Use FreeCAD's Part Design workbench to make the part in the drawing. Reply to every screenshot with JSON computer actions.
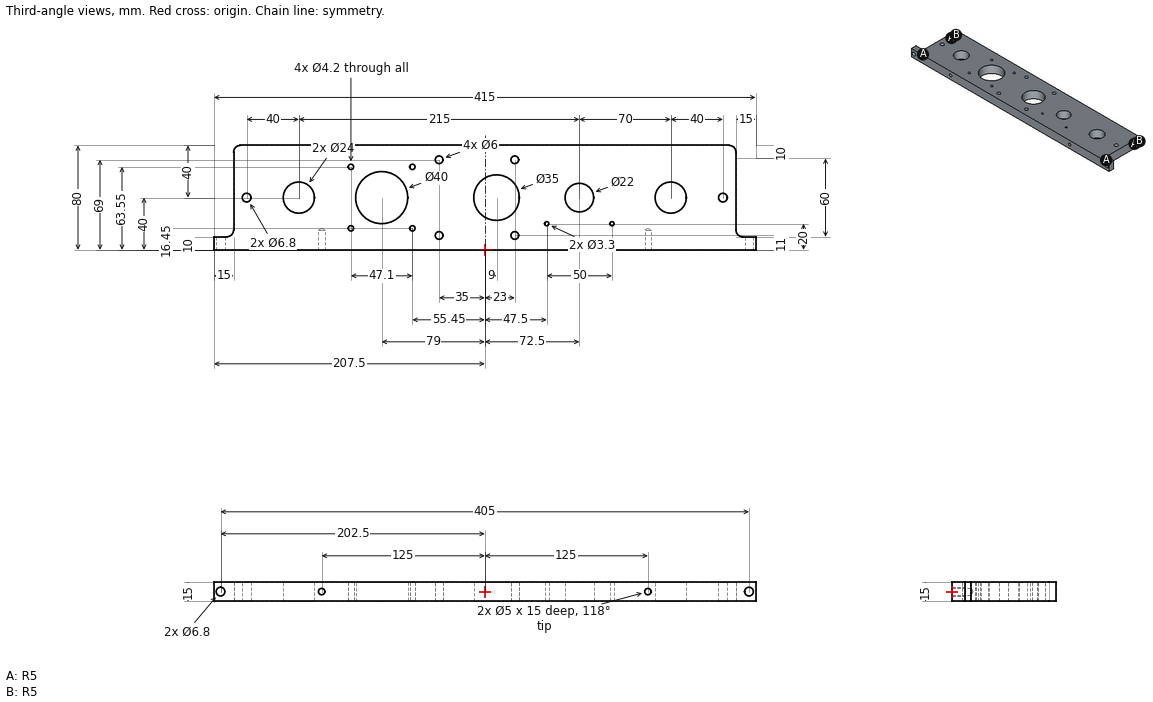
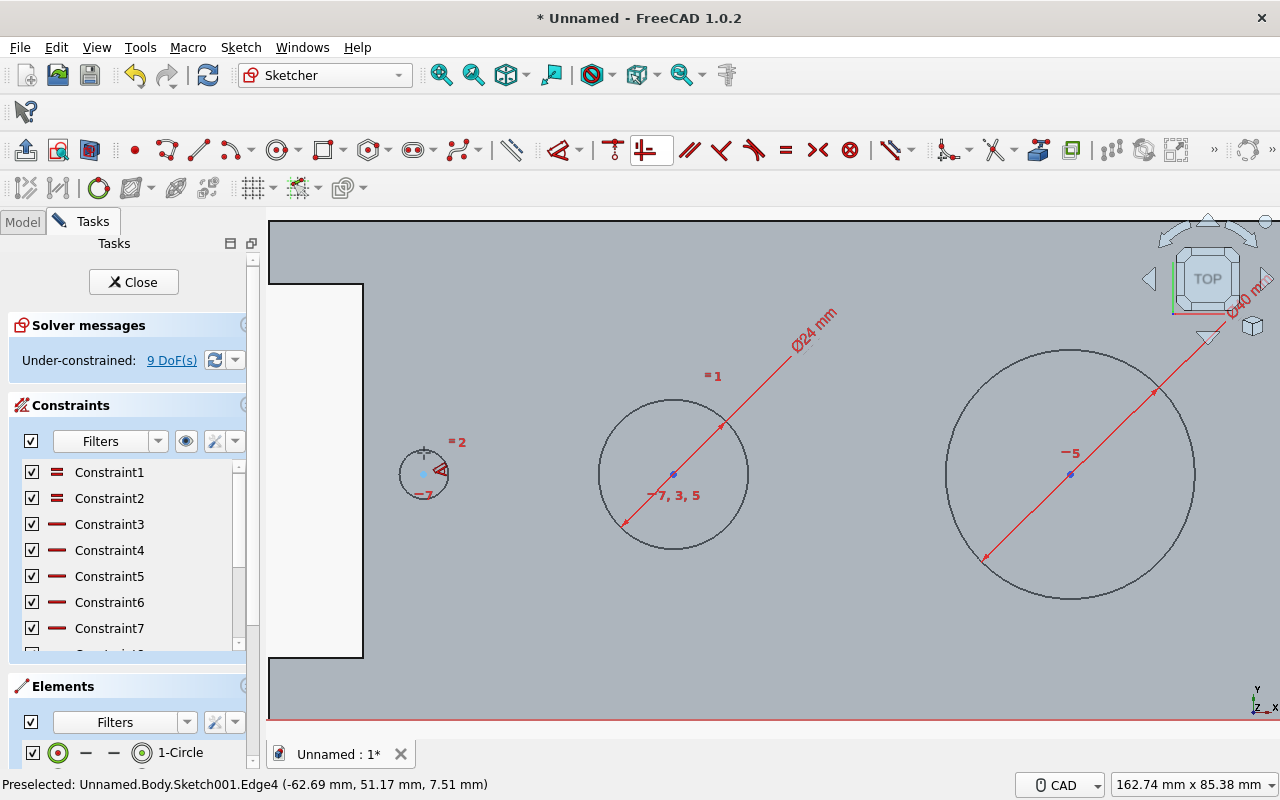
{"action": "left_click", "coordinate": [425, 450]}
{"action": "left_click", "coordinate": [426, 418]}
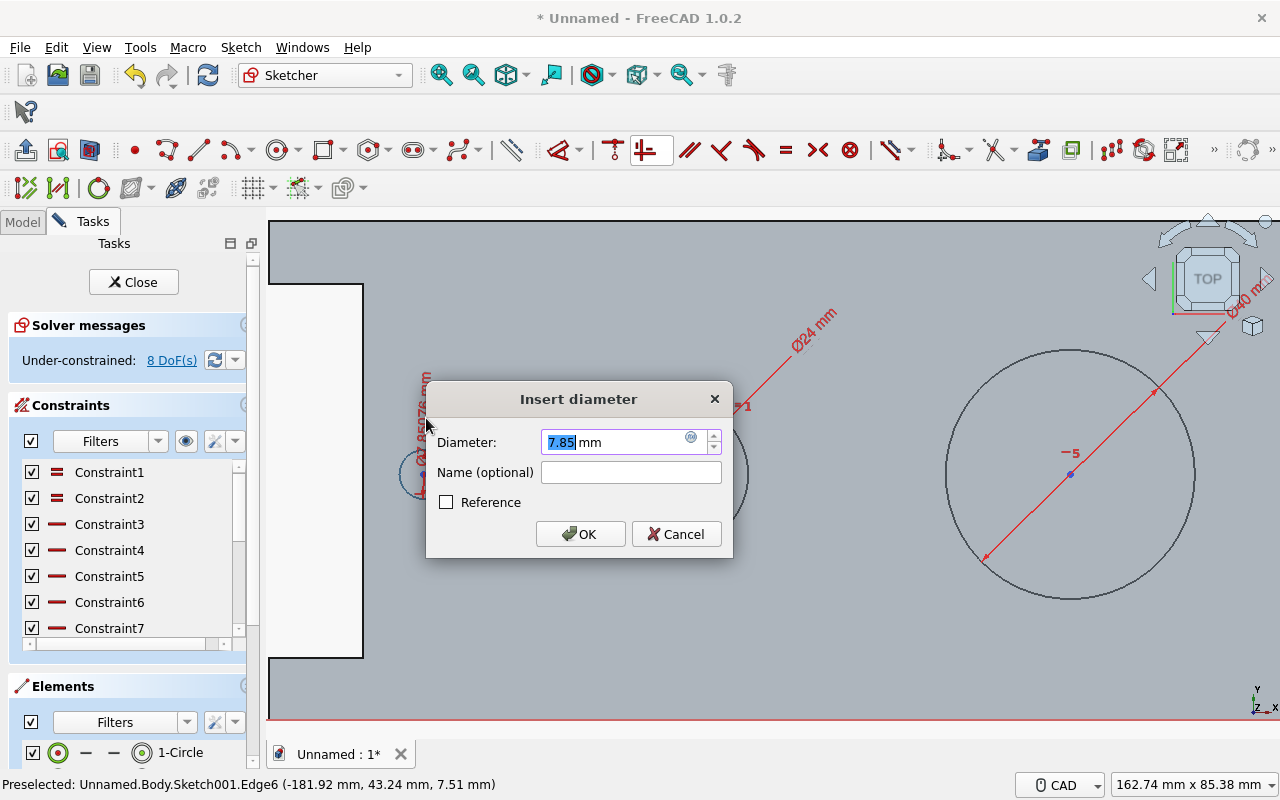
{"action": "type", "text": "6.8"}
{"action": "key", "text": "Return"}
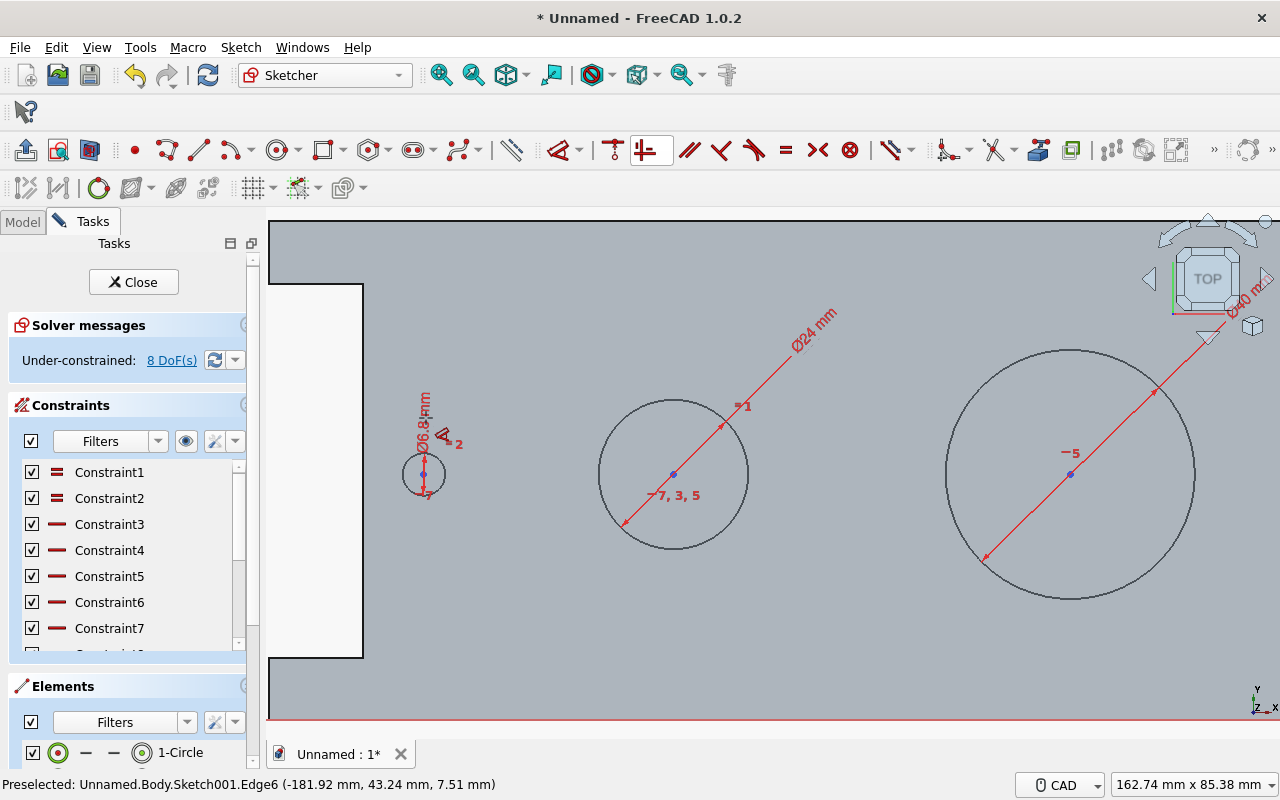
{"action": "scroll", "coordinate": [424, 453], "scroll_direction": "down", "scroll_amount": 7}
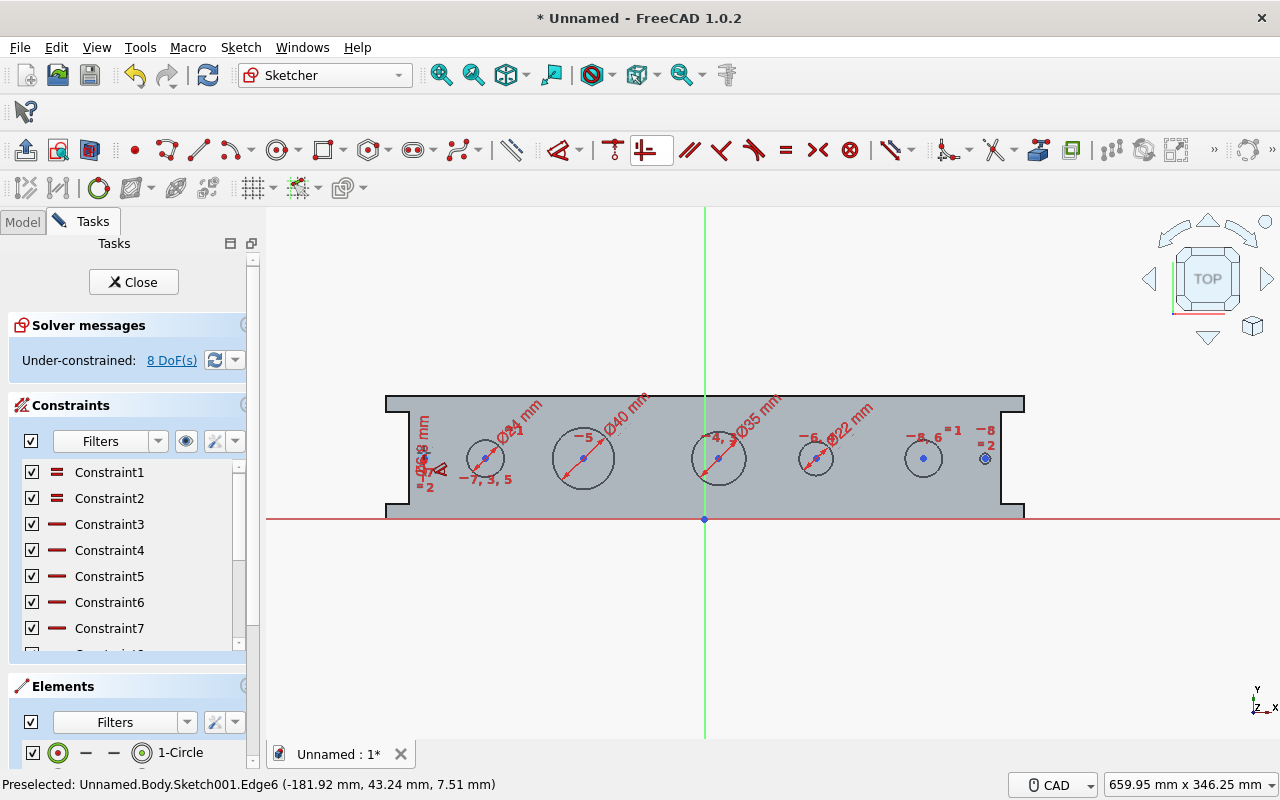
{"action": "scroll", "coordinate": [719, 459], "scroll_direction": "up", "scroll_amount": 6}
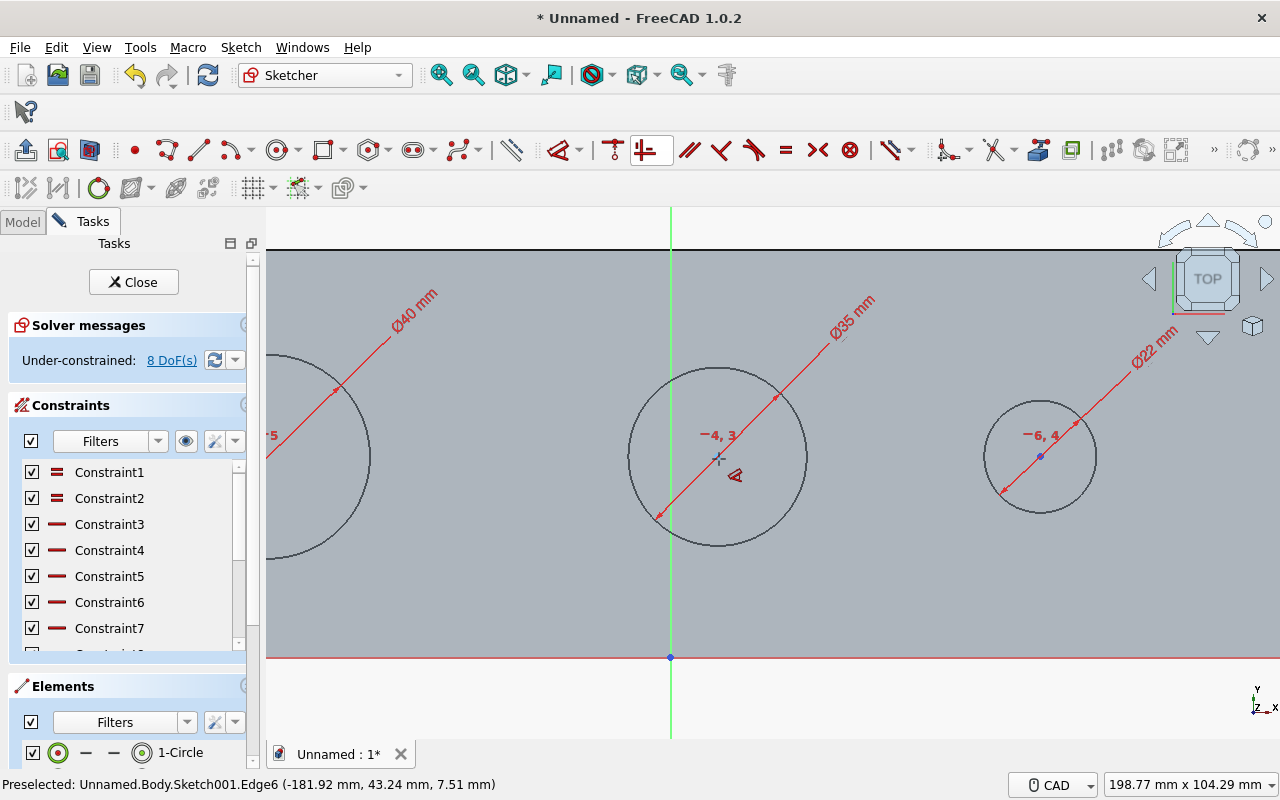
{"action": "left_click", "coordinate": [718, 457]}
{"action": "left_click", "coordinate": [694, 692]}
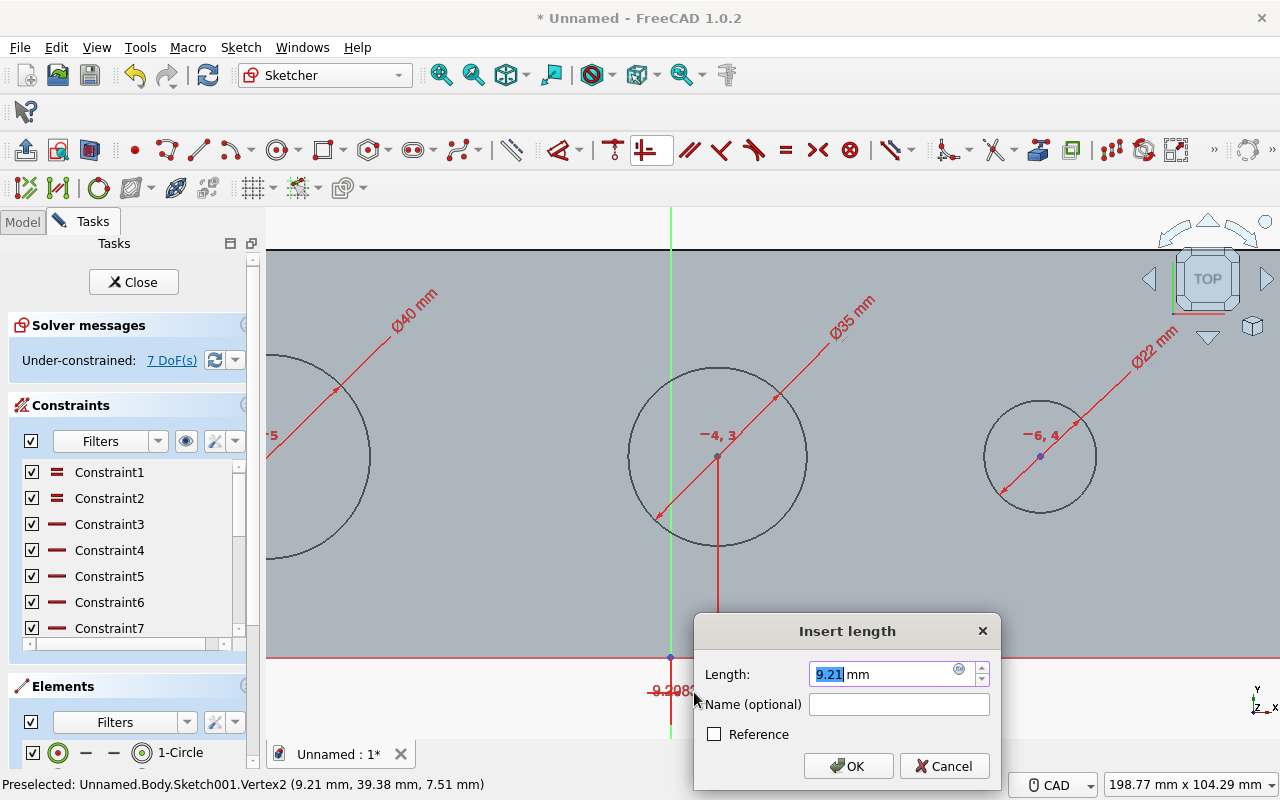
{"action": "type", "text": "9"}
{"action": "key", "text": "Return"}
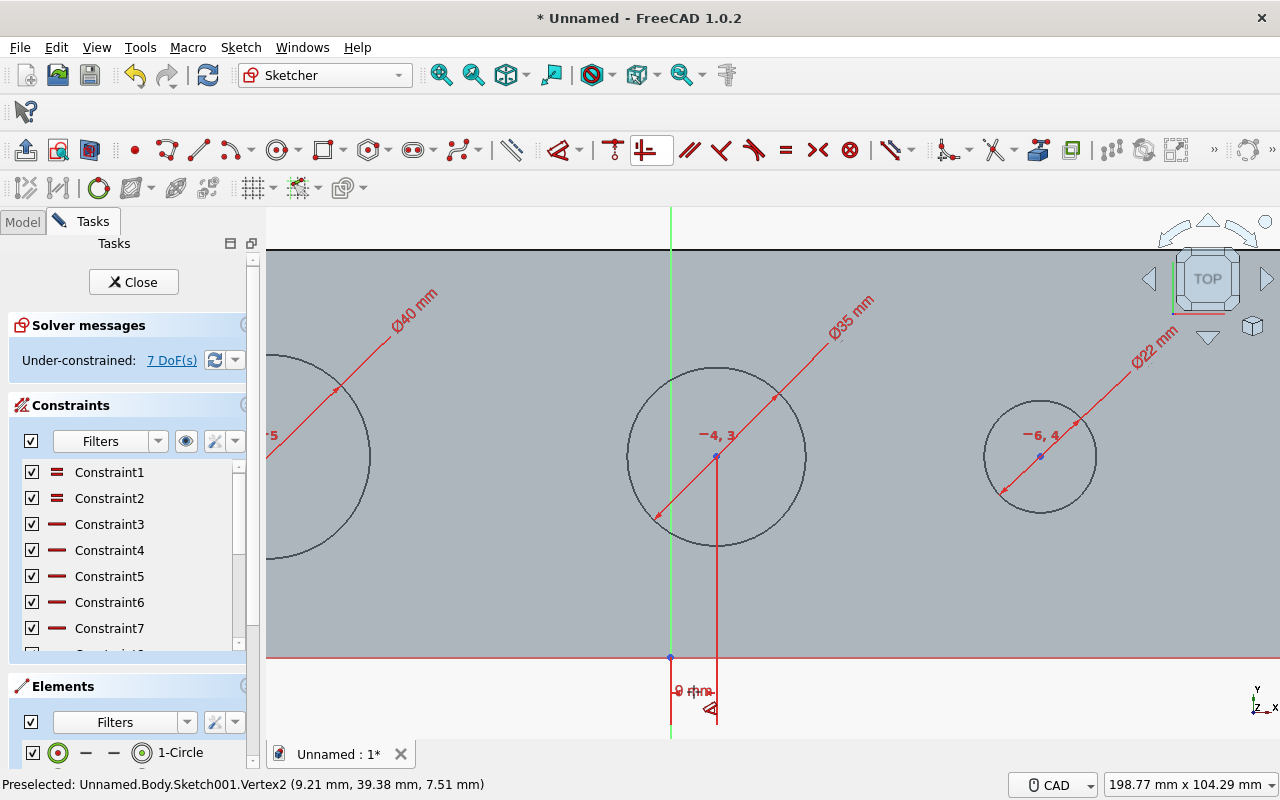
{"action": "scroll", "coordinate": [719, 459], "scroll_direction": "down", "scroll_amount": 6}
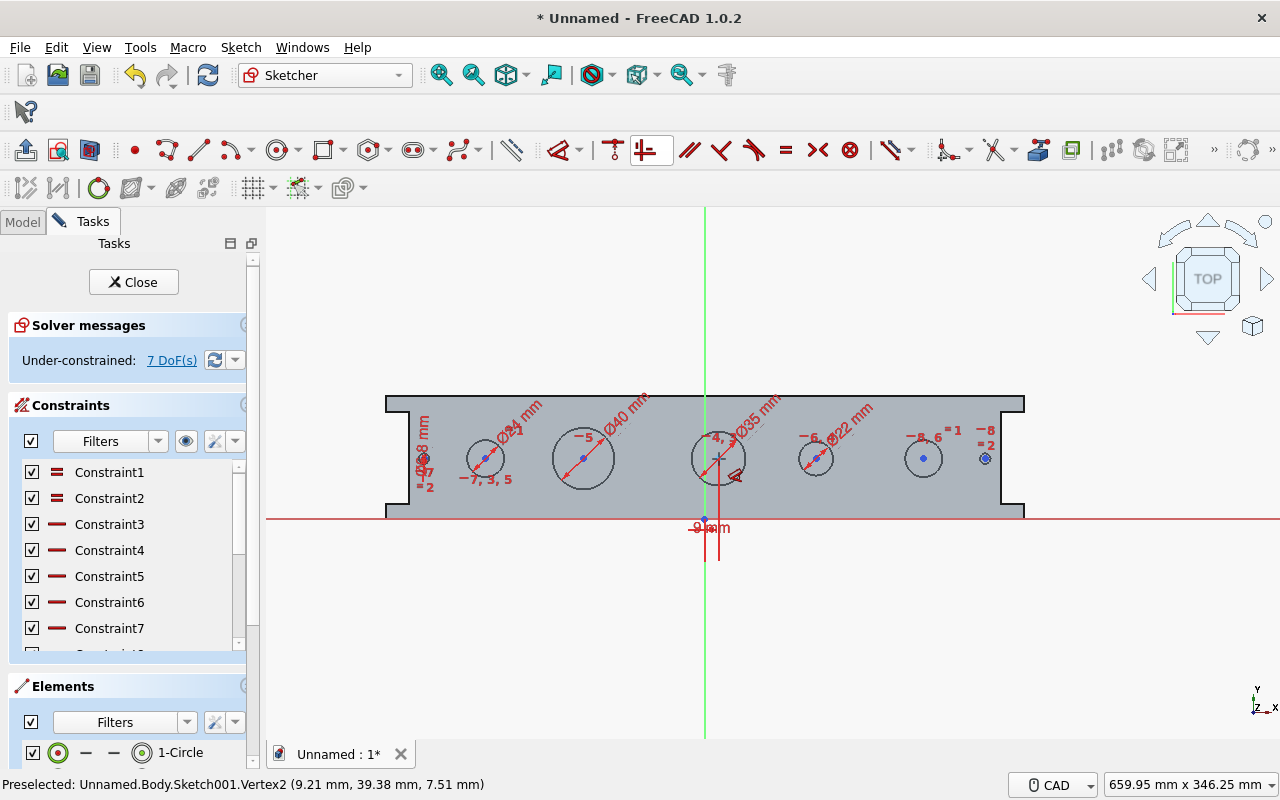
{"action": "left_click", "coordinate": [486, 459]}
{"action": "left_click", "coordinate": [452, 489]}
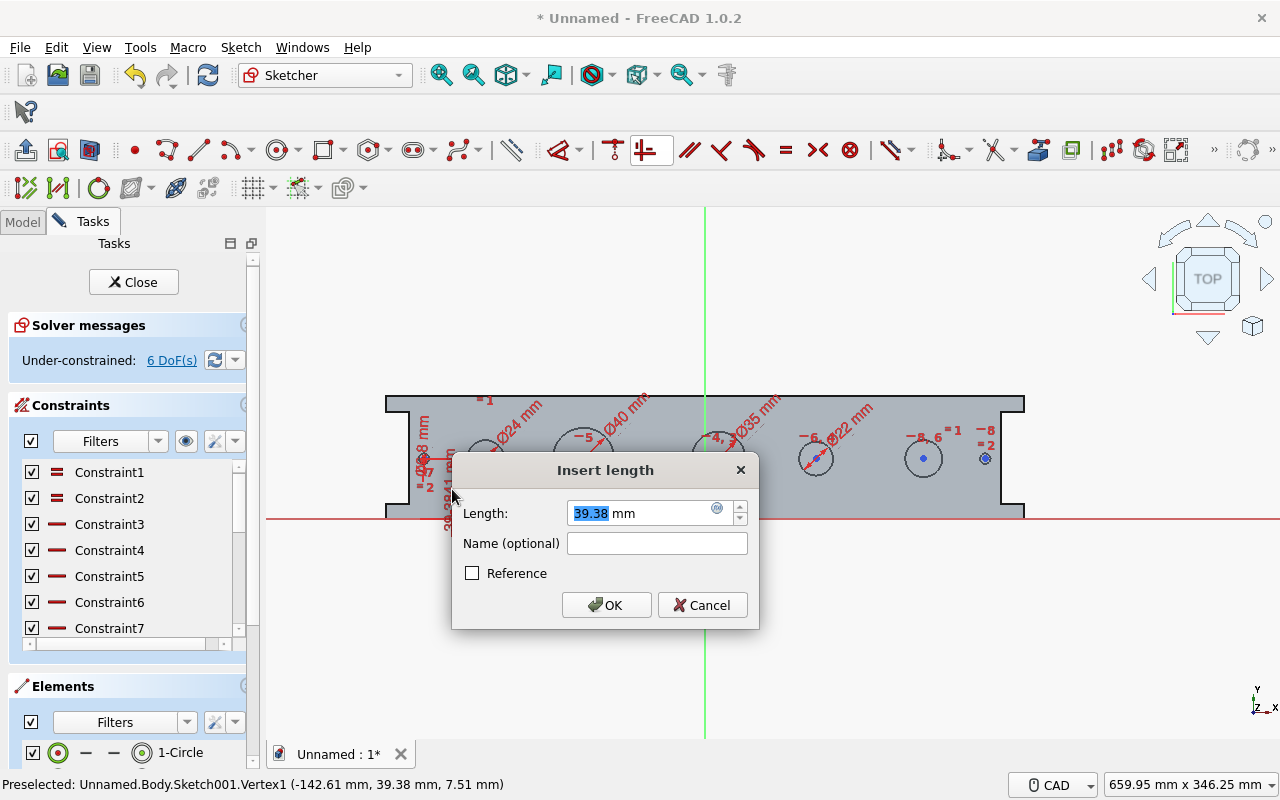
{"action": "type", "text": "40"}
{"action": "key", "text": "Return"}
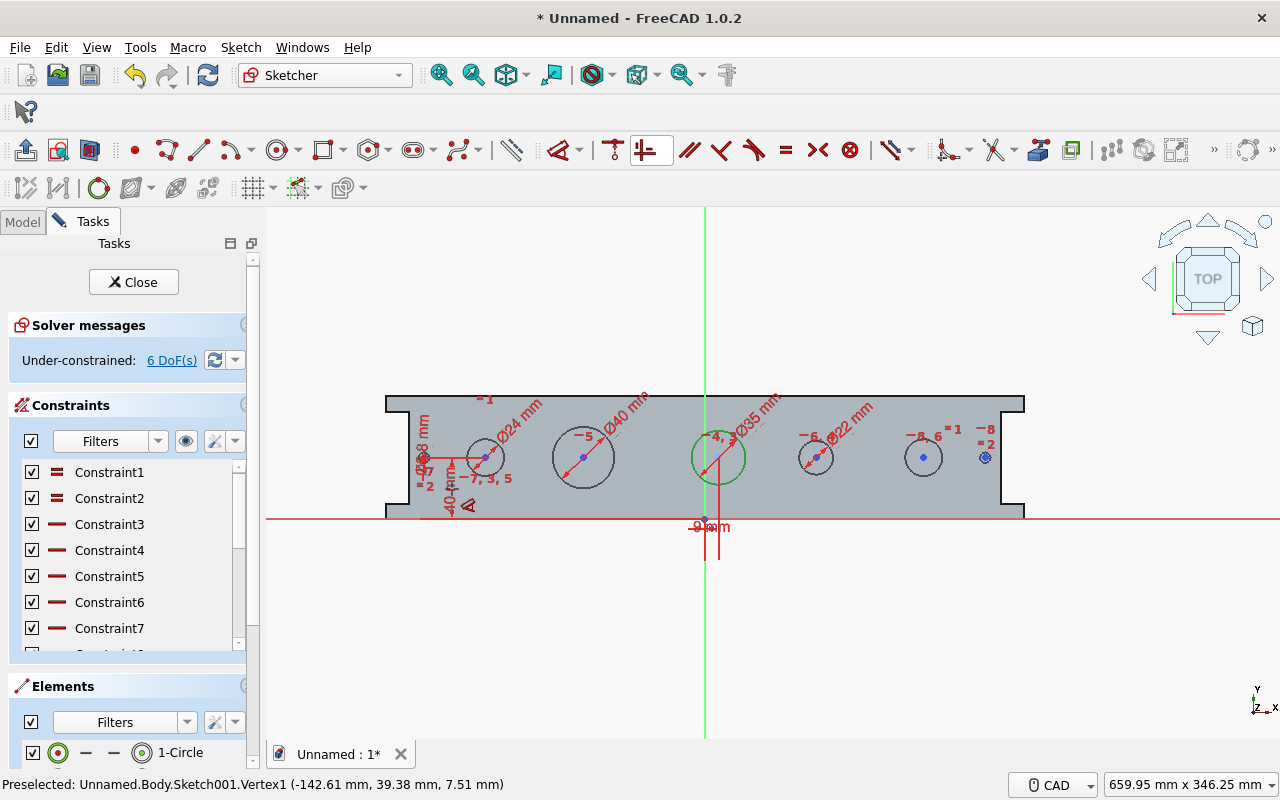
{"action": "left_click", "coordinate": [583, 458]}
{"action": "left_click", "coordinate": [644, 553]}